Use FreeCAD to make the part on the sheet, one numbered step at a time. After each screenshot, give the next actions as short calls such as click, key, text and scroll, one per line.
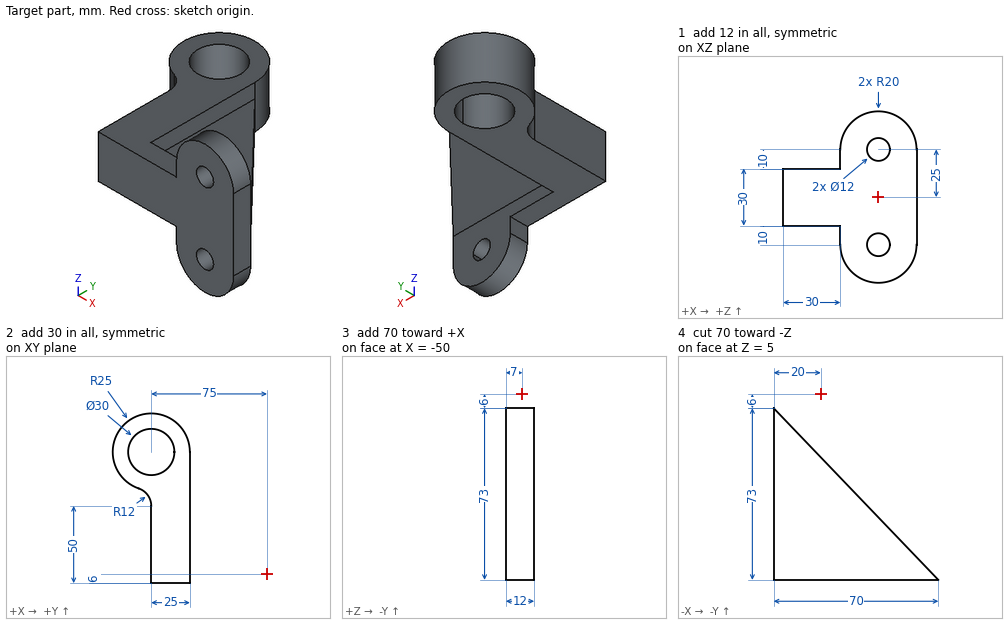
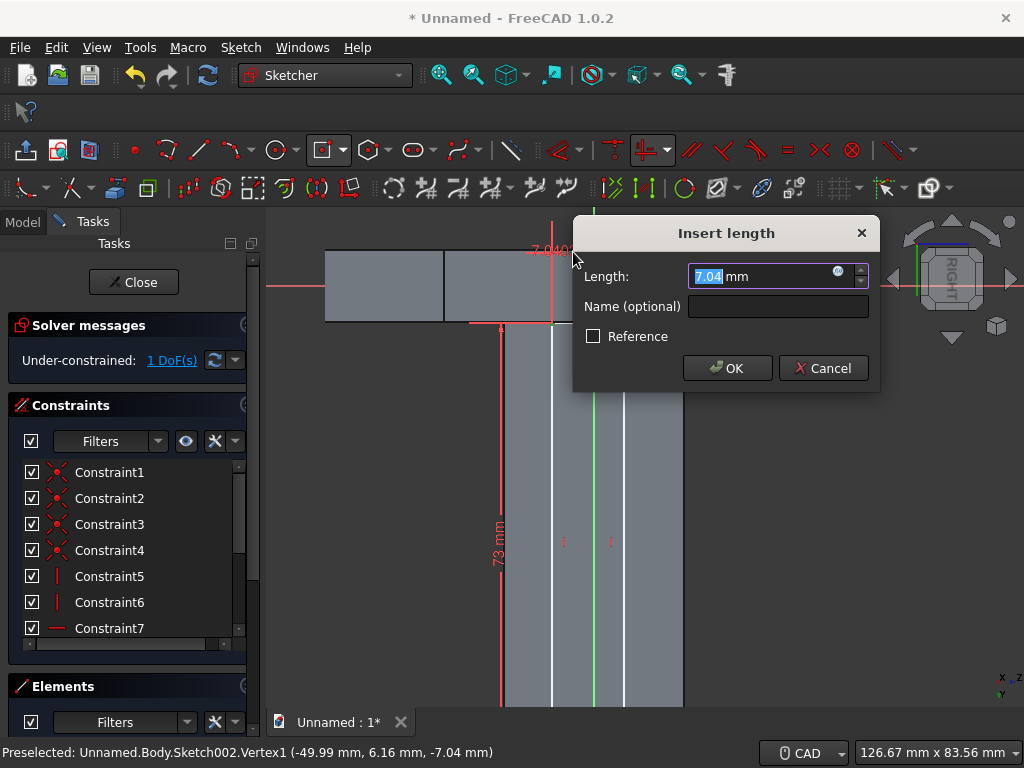
text(7)
key(Return)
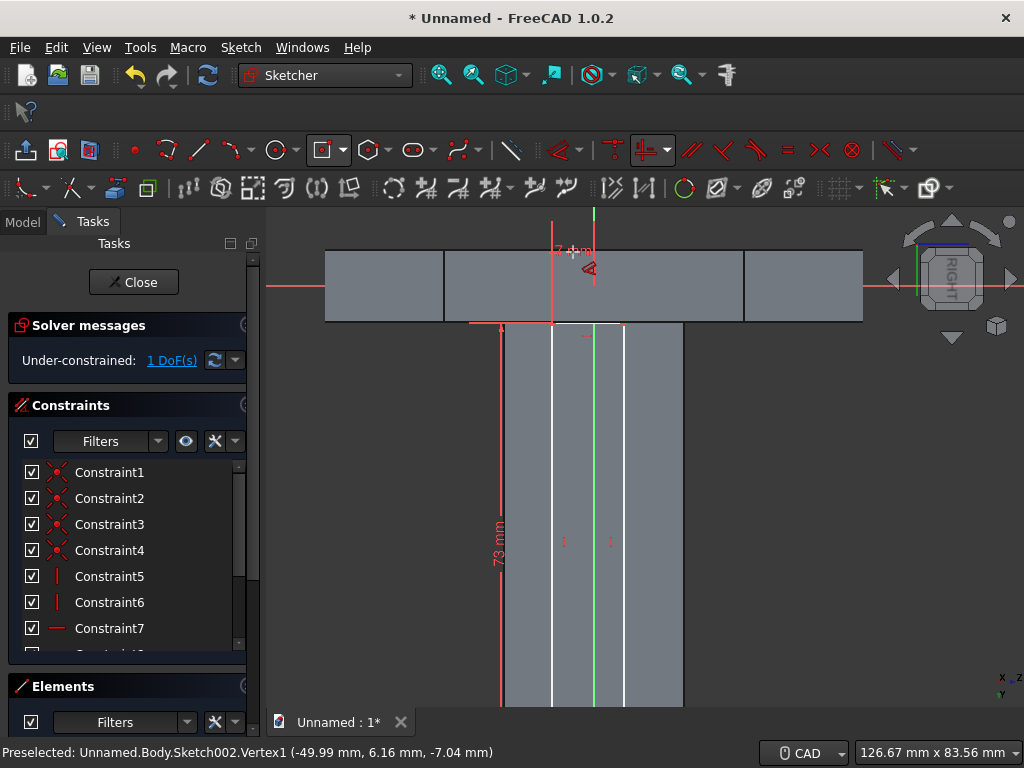
click(552, 323)
click(518, 304)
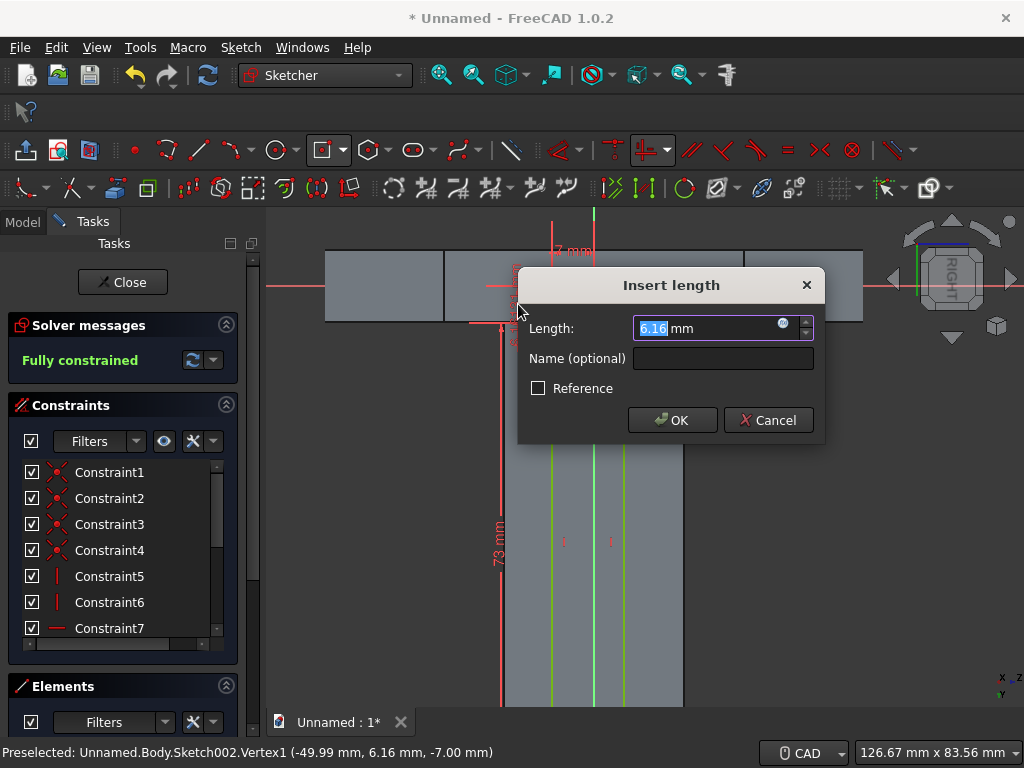
text(6)
key(Return)
key(Escape)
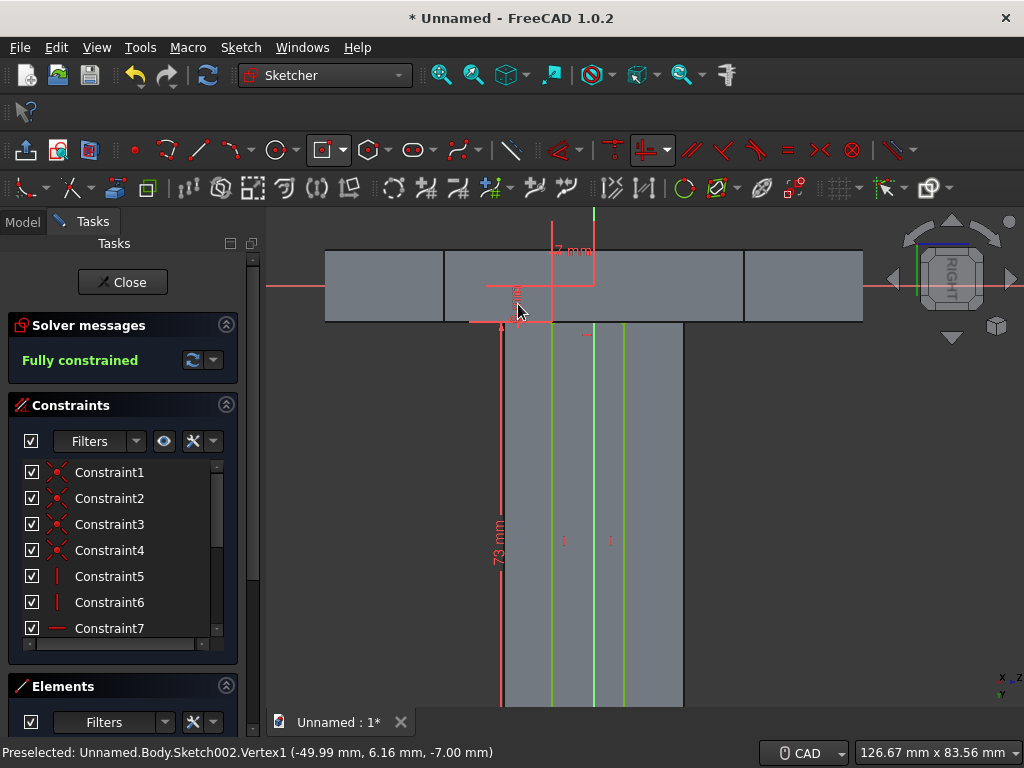
click(123, 282)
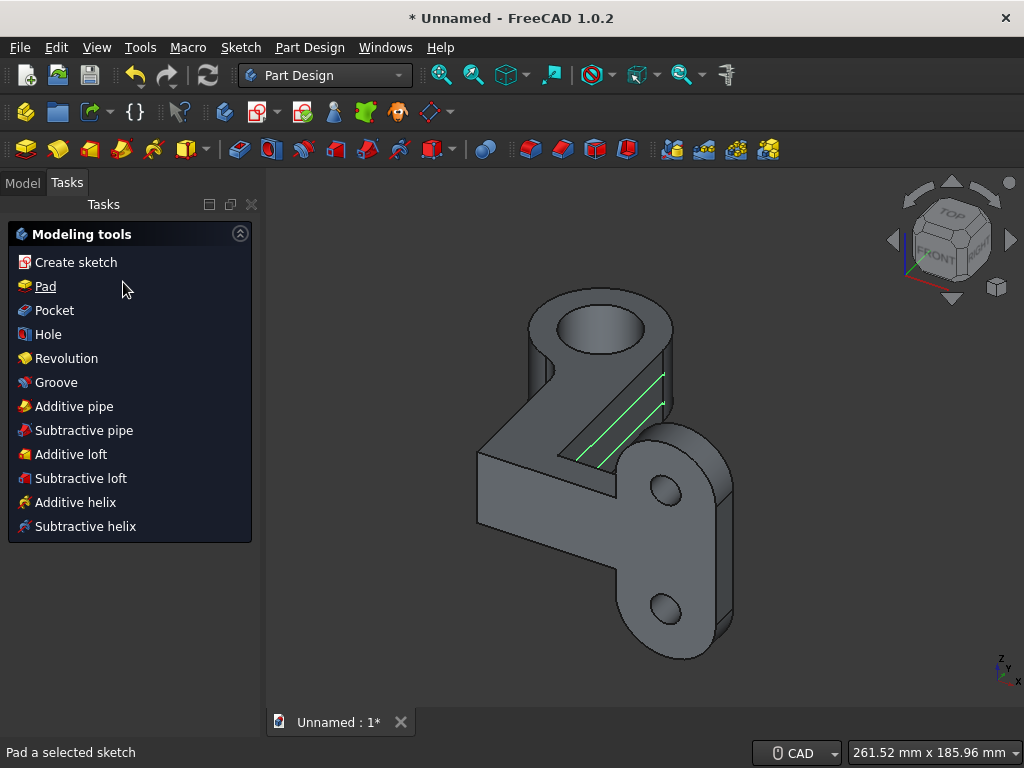
click(26, 150)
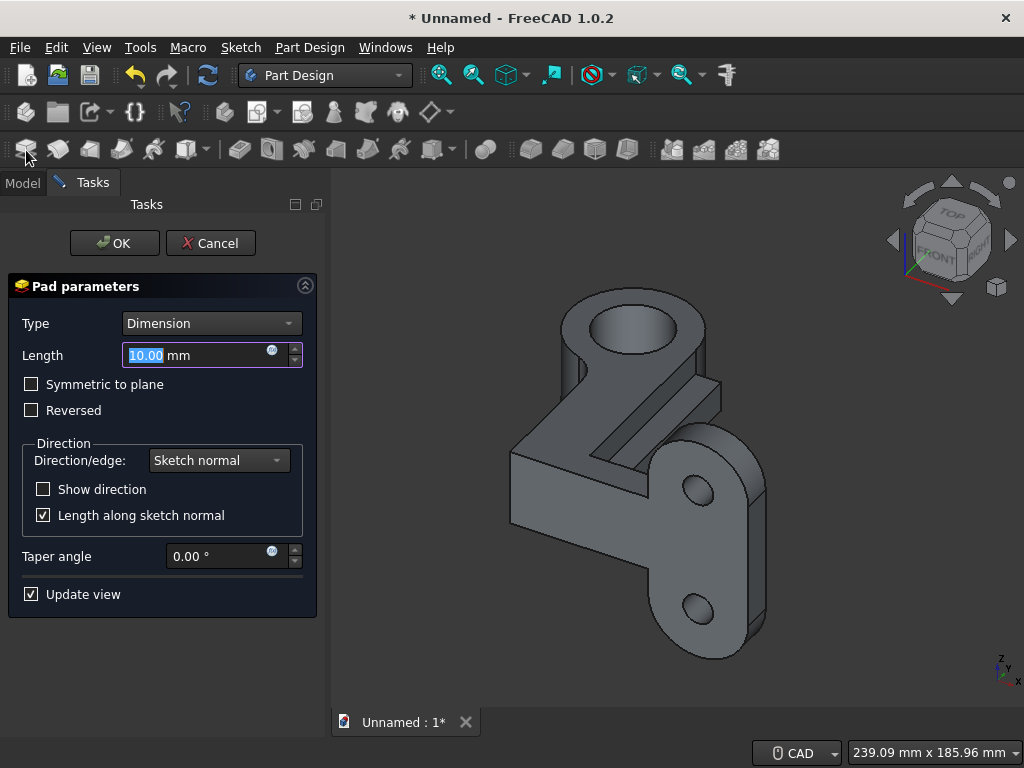
text(70)
key(Tab)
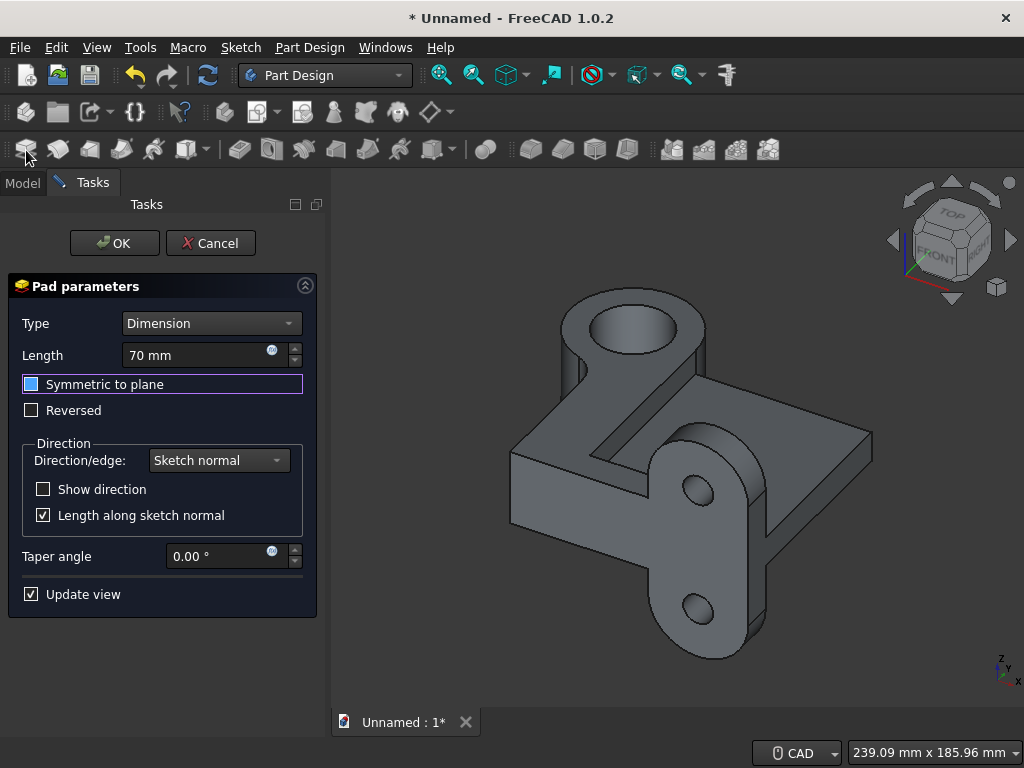
click(115, 243)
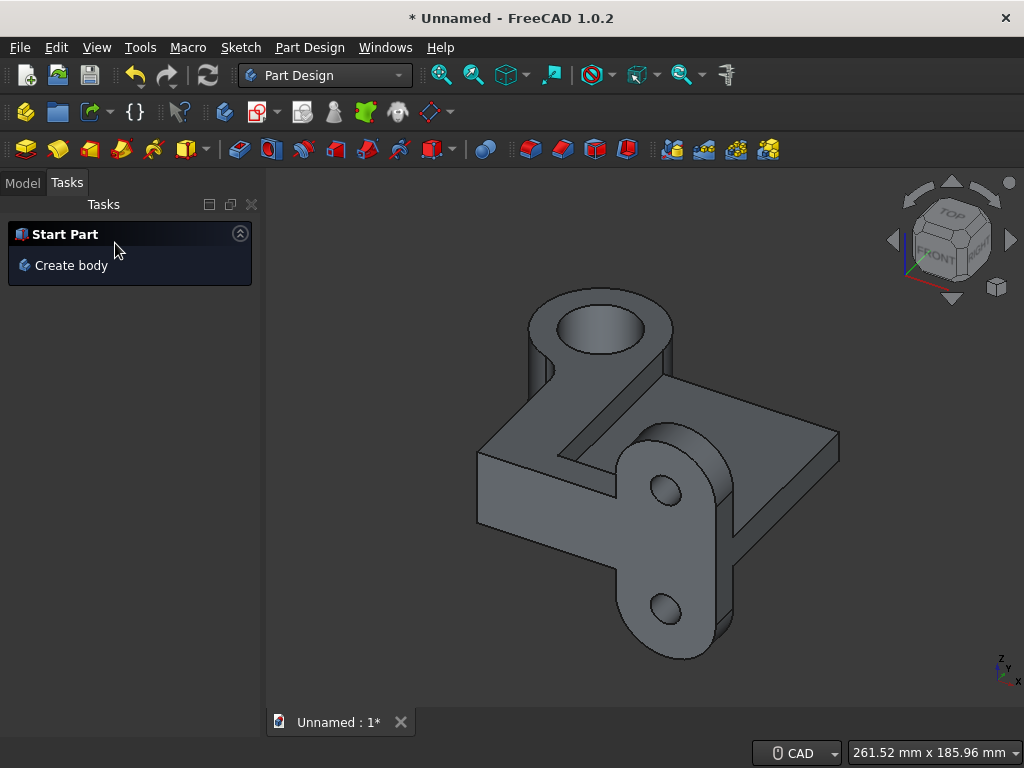
click(739, 448)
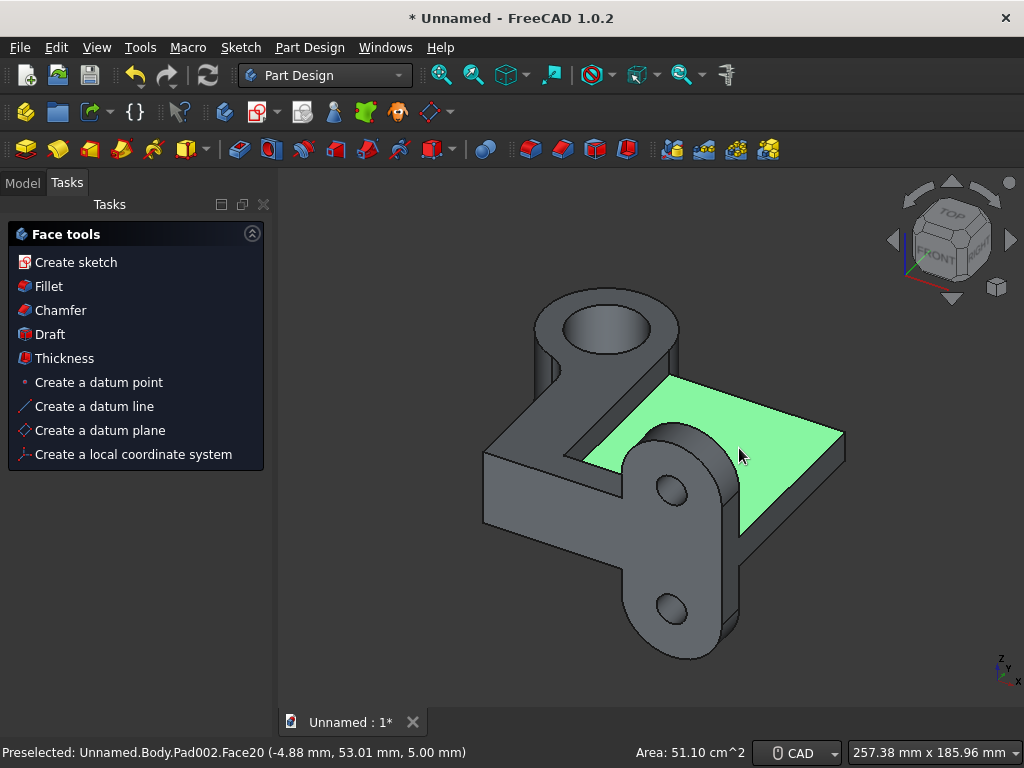
click(258, 112)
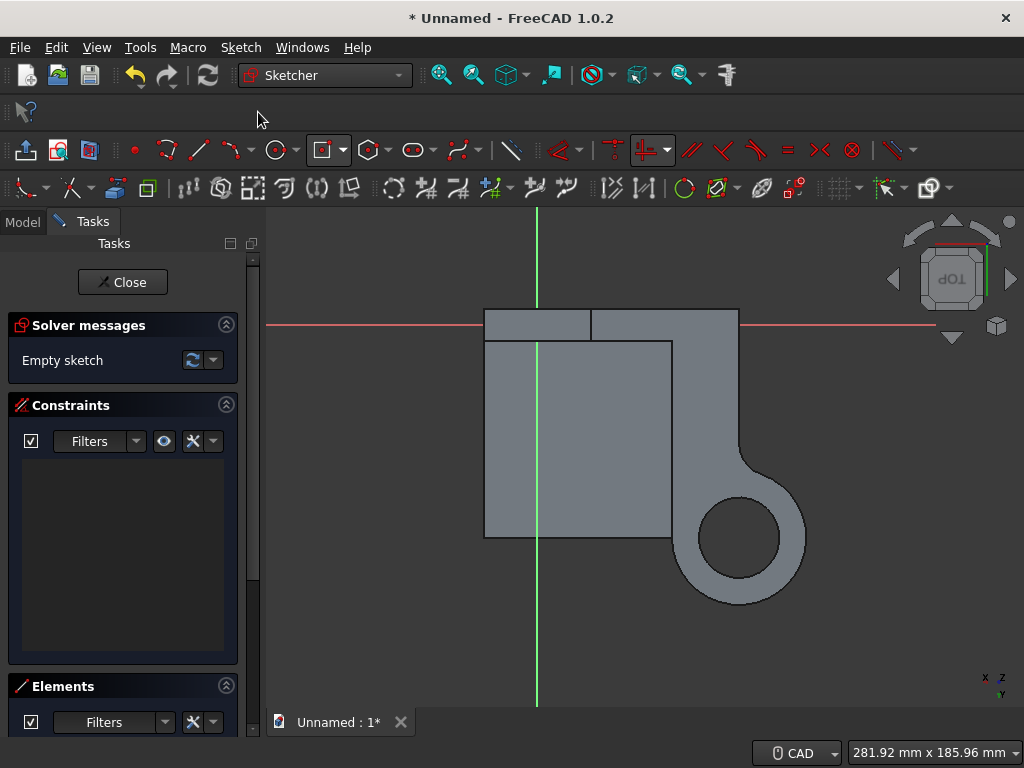
scroll(580, 380, up, 2)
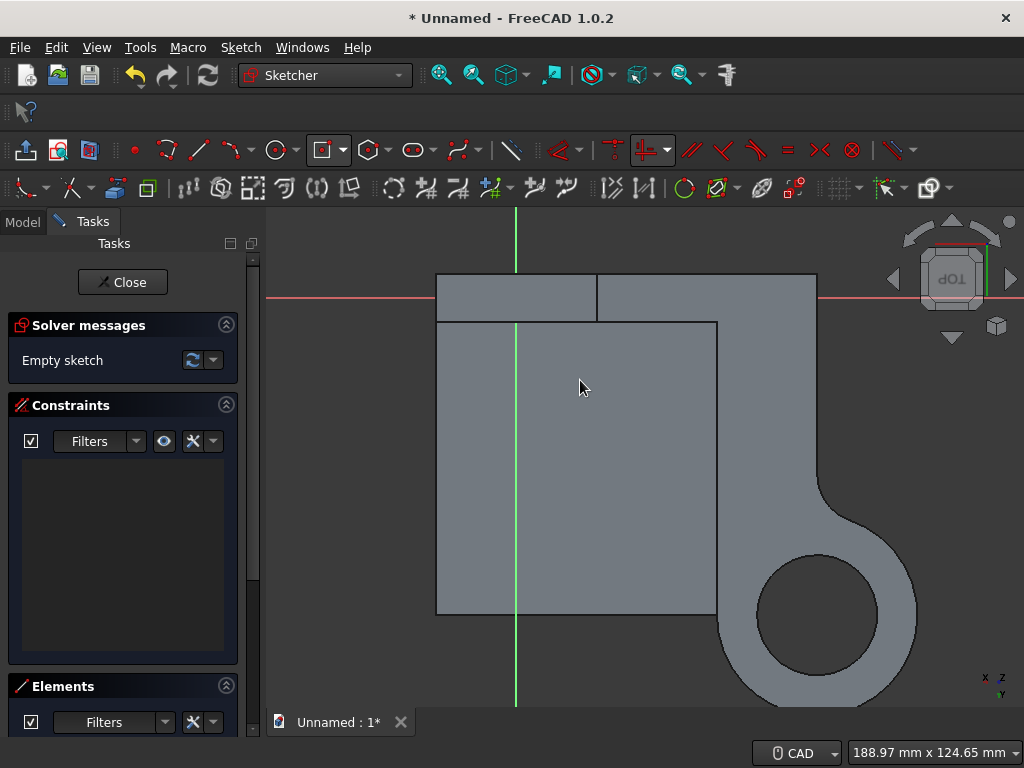
click(168, 150)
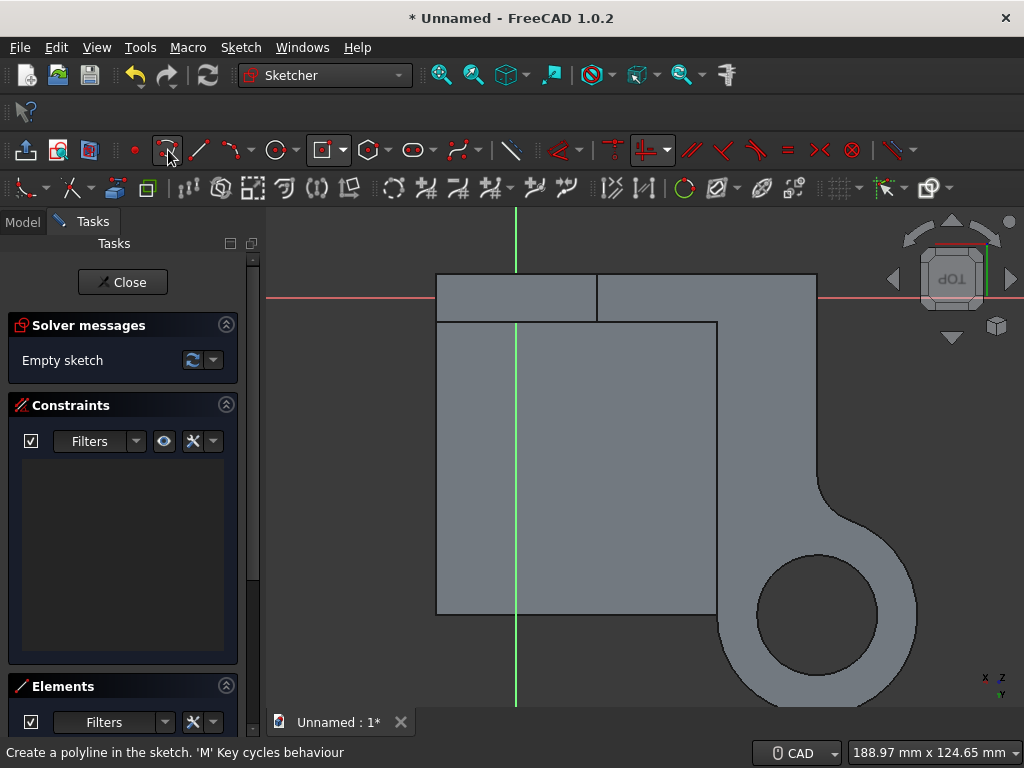
click(436, 322)
click(436, 615)
click(717, 615)
click(436, 323)
key(Escape)
key(Escape)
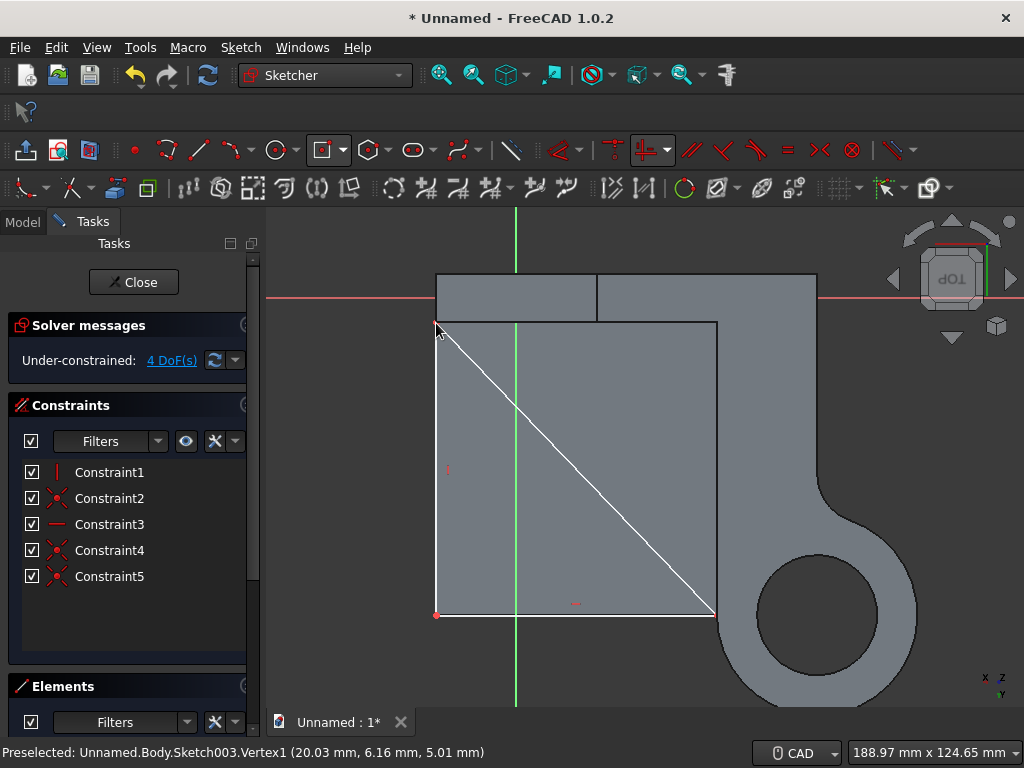
click(558, 150)